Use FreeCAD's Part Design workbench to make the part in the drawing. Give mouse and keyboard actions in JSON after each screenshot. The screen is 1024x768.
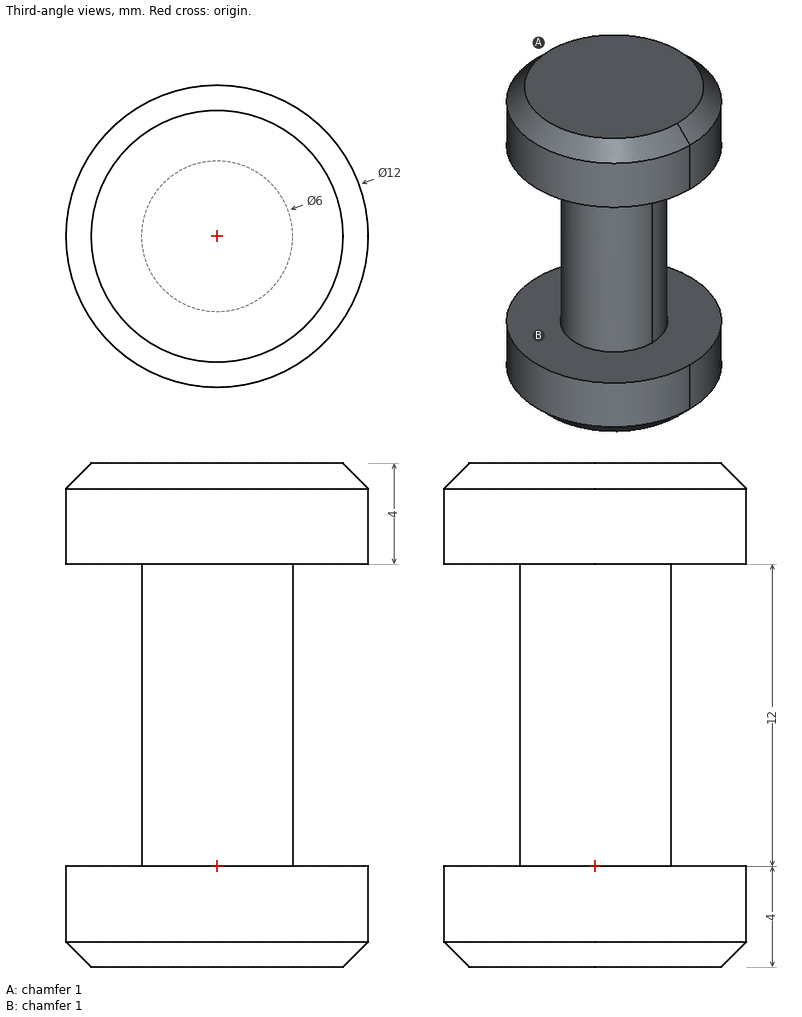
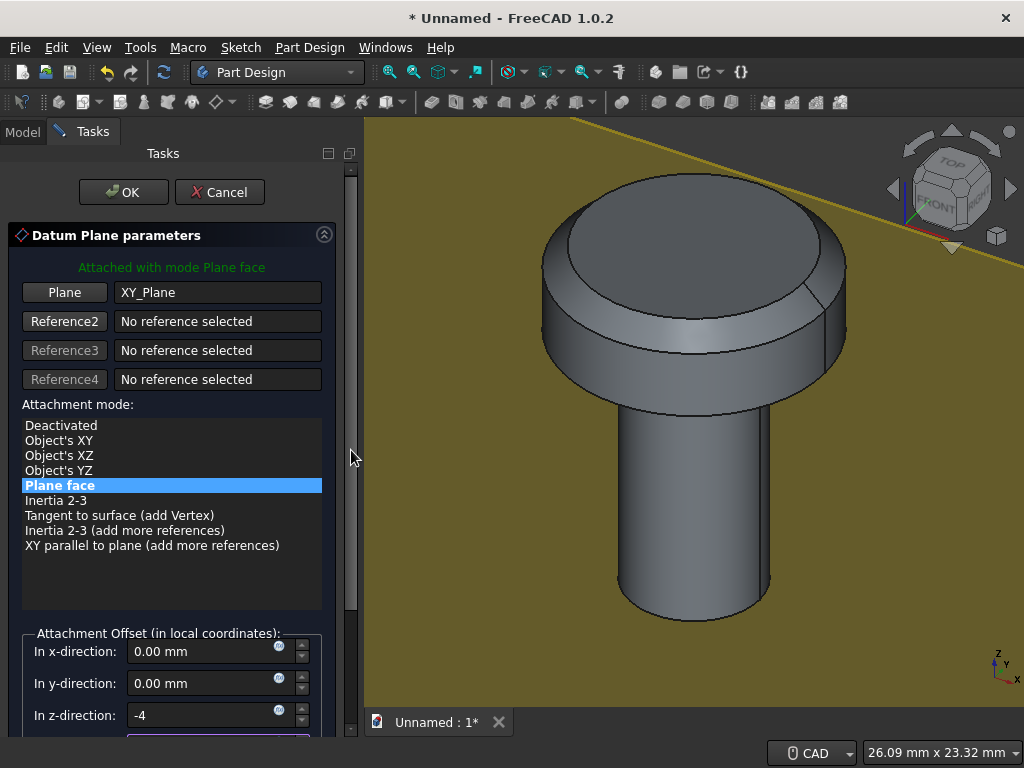
{"action": "left_click", "coordinate": [124, 192]}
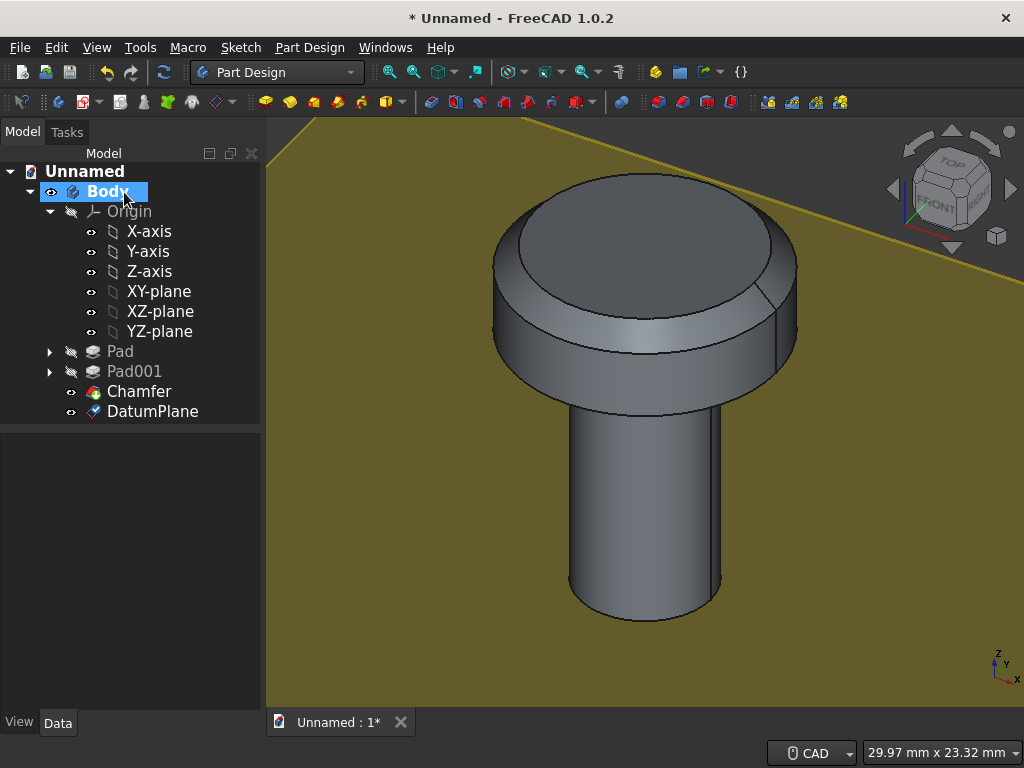
{"action": "left_click", "coordinate": [116, 412]}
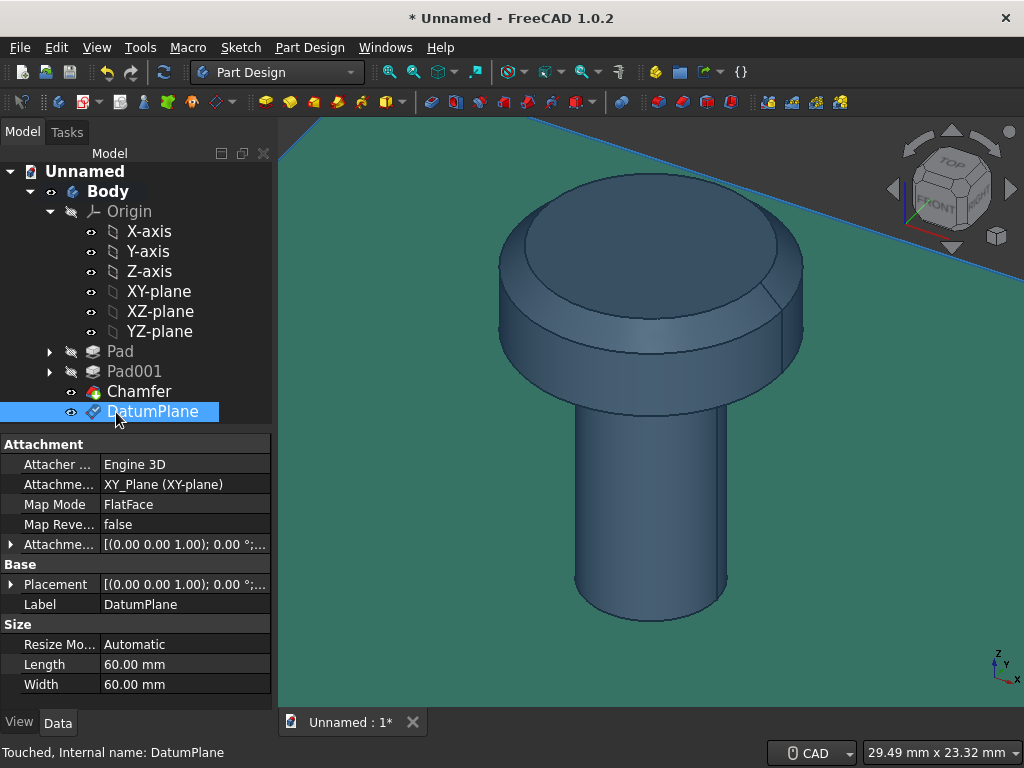
{"action": "left_click", "coordinate": [84, 102]}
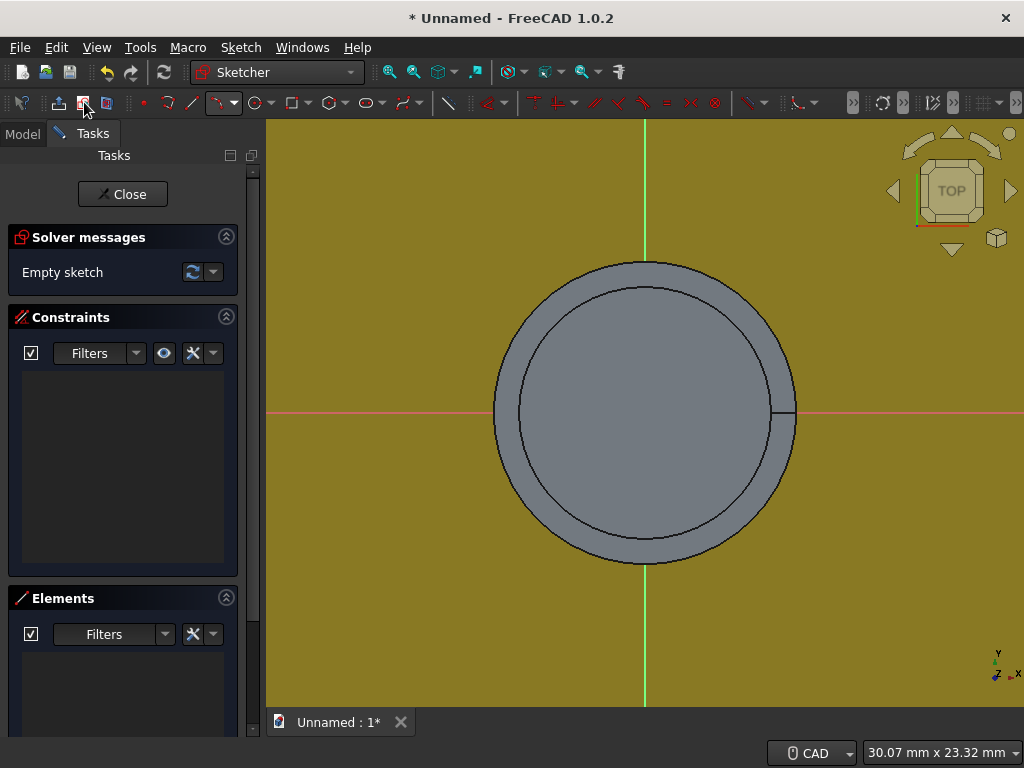
{"action": "key", "text": "q s"}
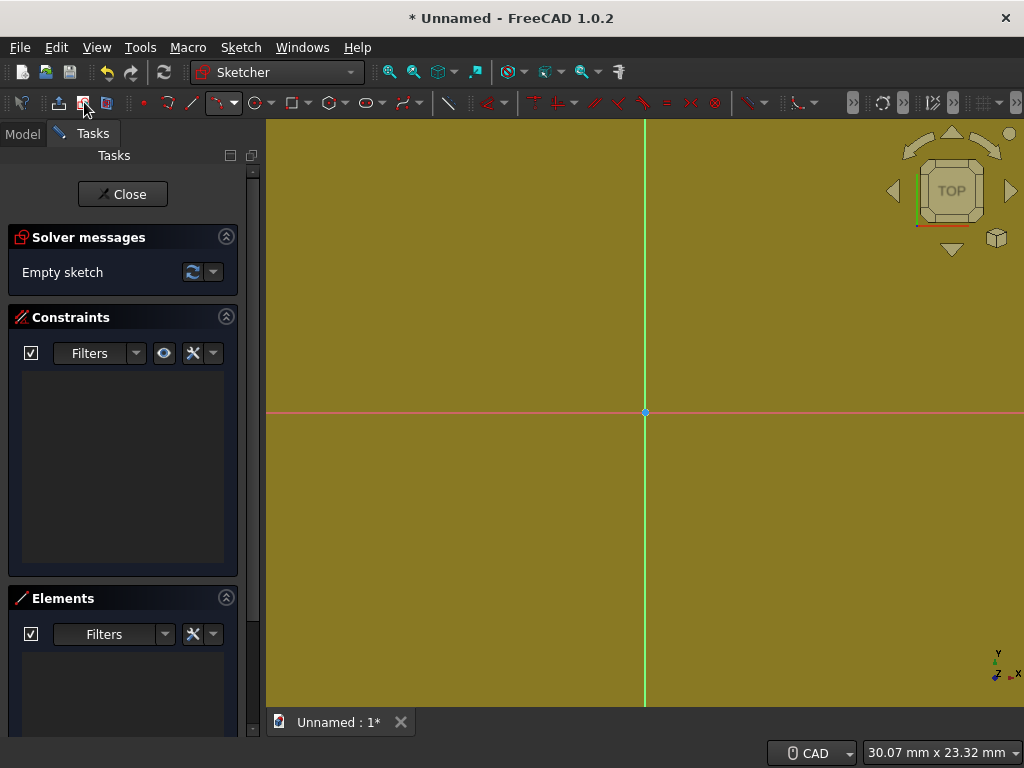
{"action": "key", "text": "g c"}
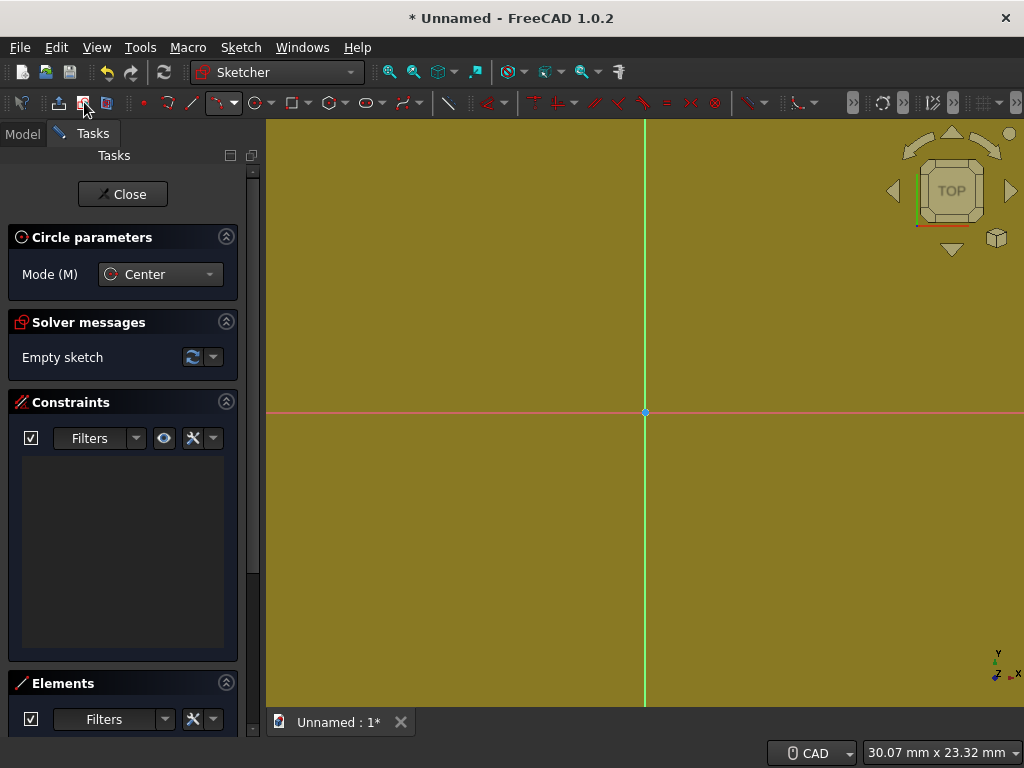
{"action": "left_click", "coordinate": [645, 413]}
{"action": "left_click", "coordinate": [752, 306]}
{"action": "key", "text": "Escape"}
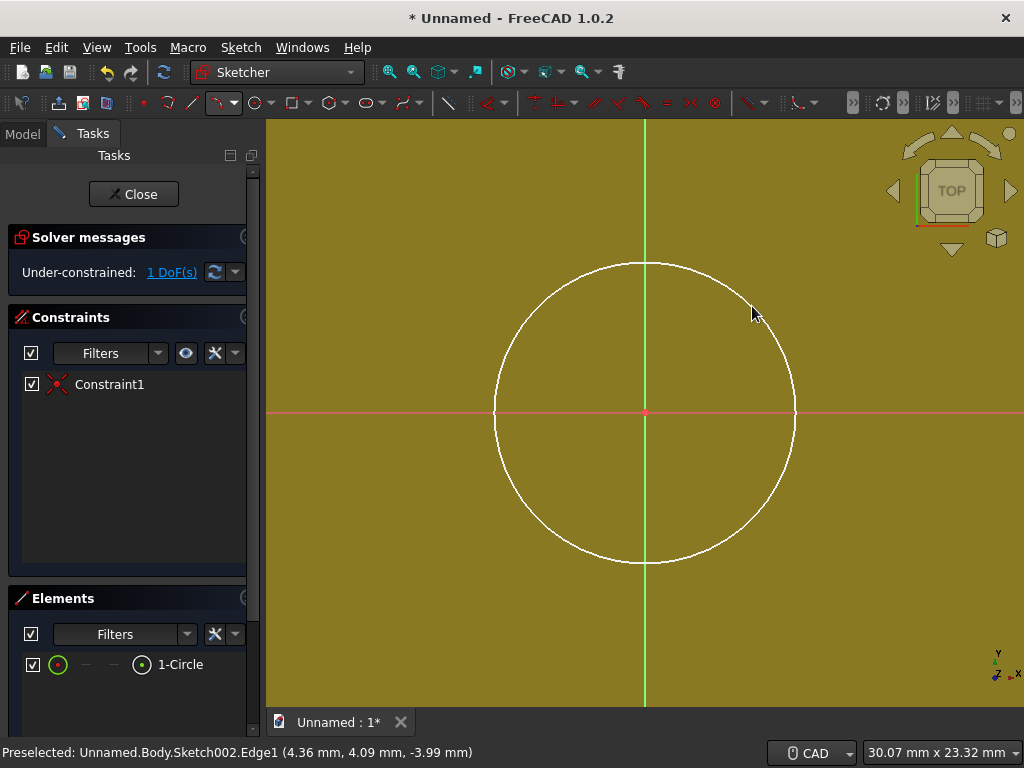
{"action": "left_click", "coordinate": [488, 104]}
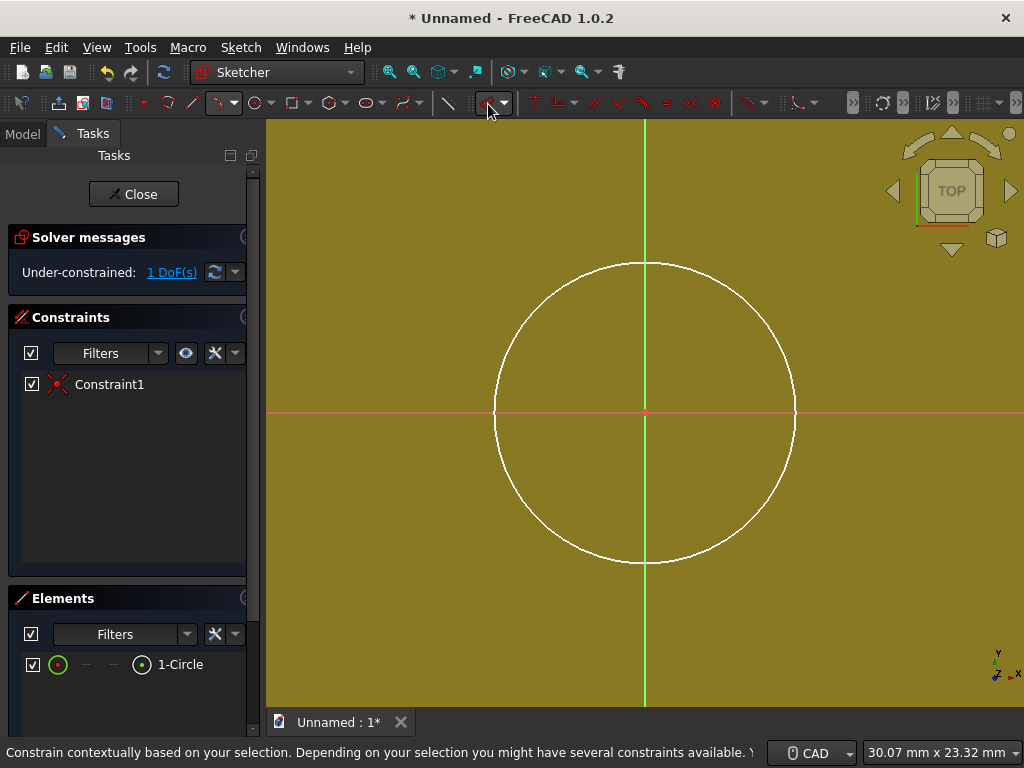
{"action": "left_click", "coordinate": [751, 306]}
{"action": "left_click", "coordinate": [774, 283]}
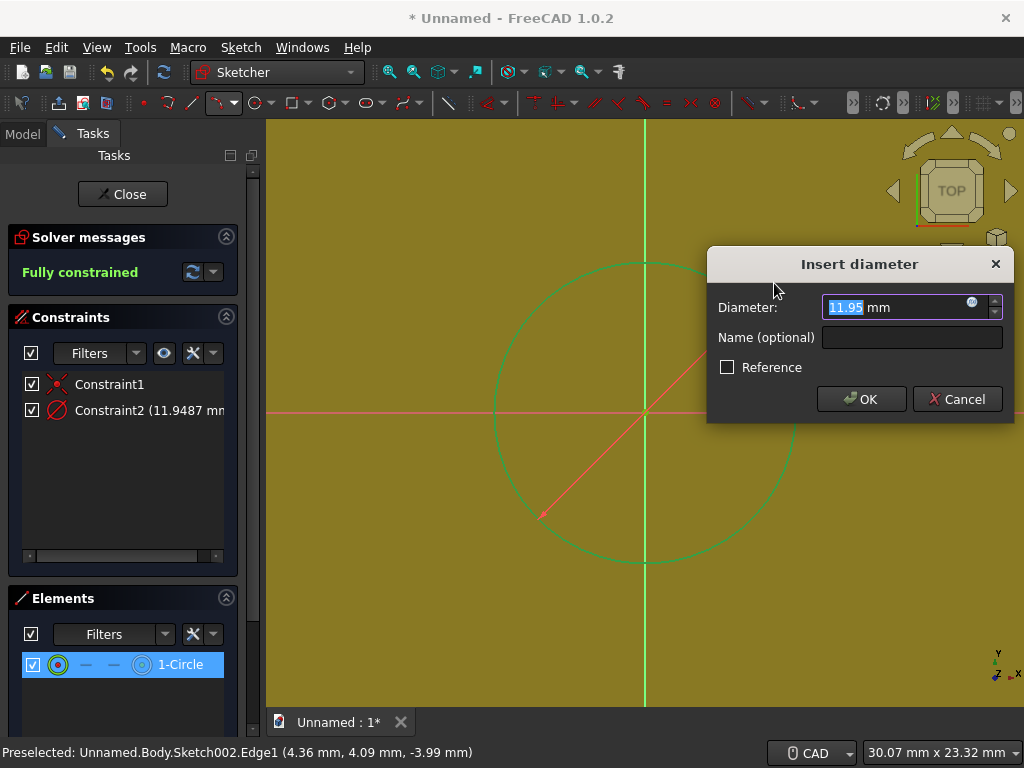
{"action": "type", "text": "12"}
{"action": "key", "text": "Return"}
{"action": "key", "text": "Escape"}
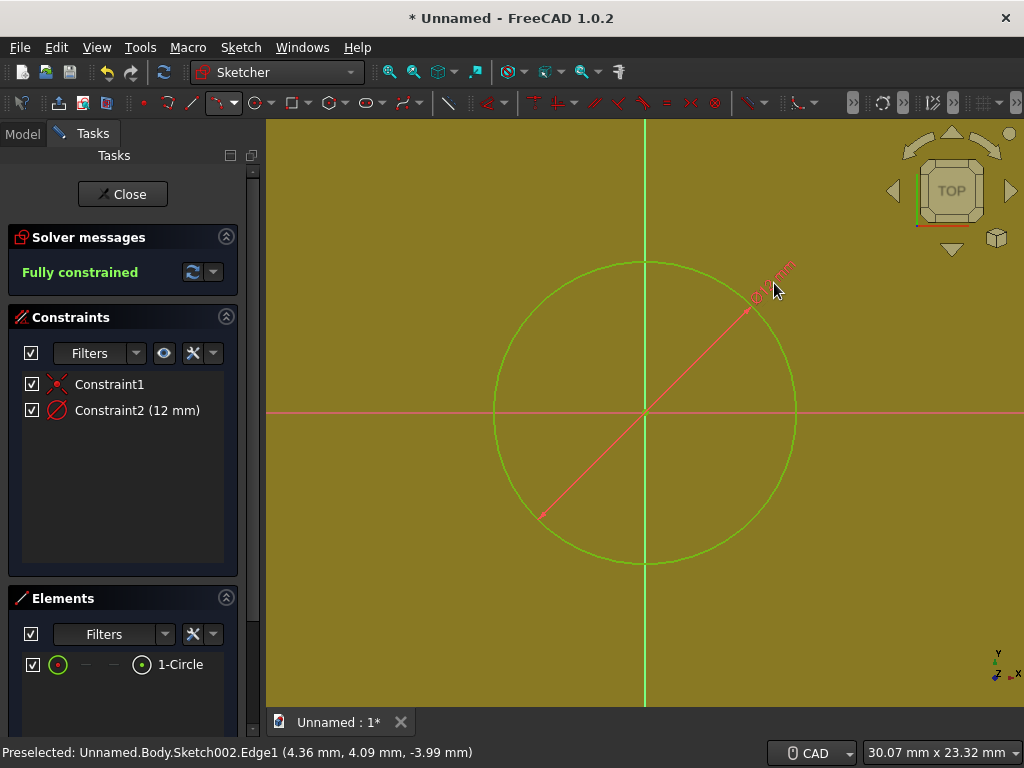
{"action": "left_click", "coordinate": [123, 194]}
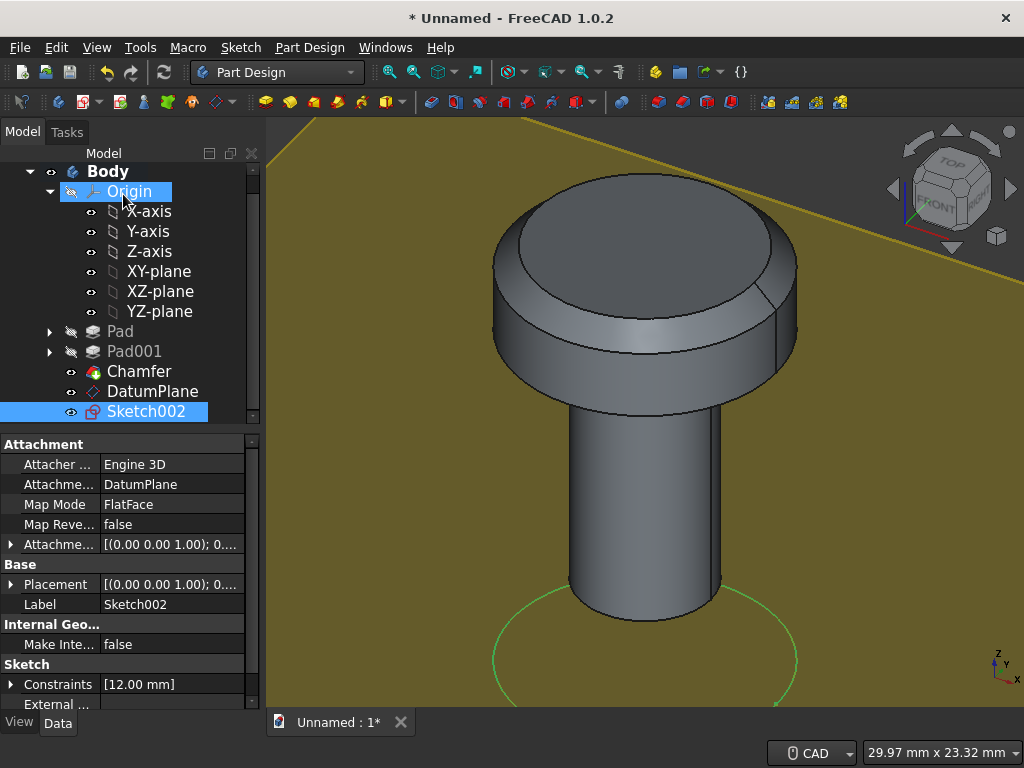
{"action": "left_click", "coordinate": [266, 102]}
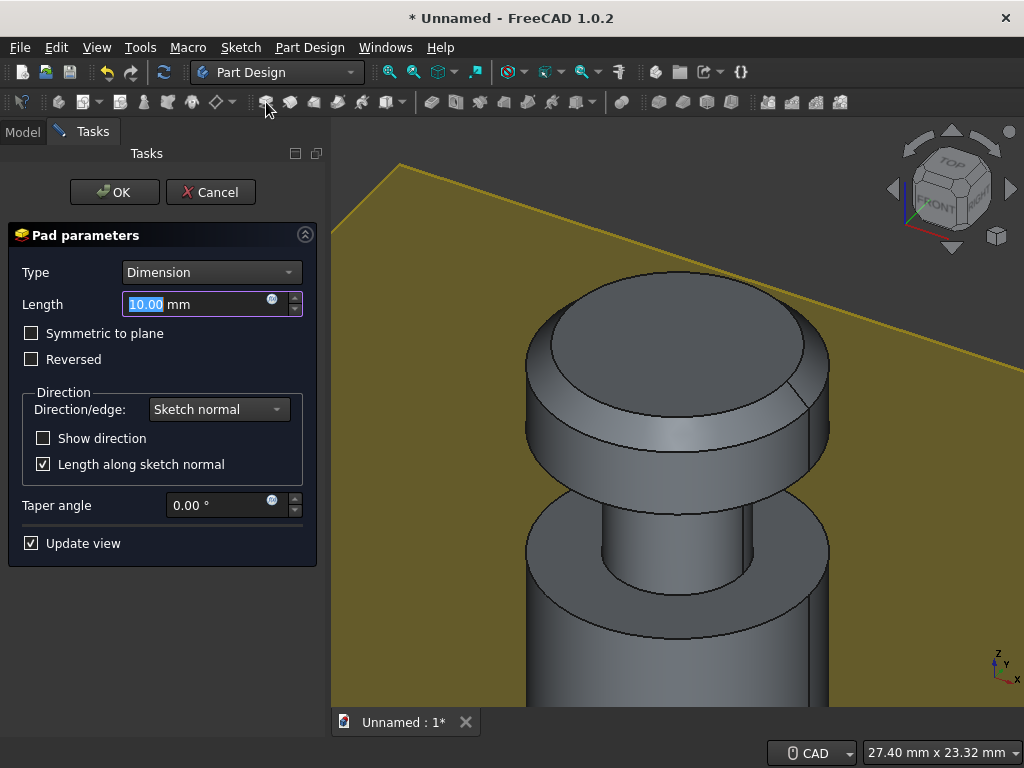
{"action": "type", "text": "4"}
{"action": "key", "text": "Tab"}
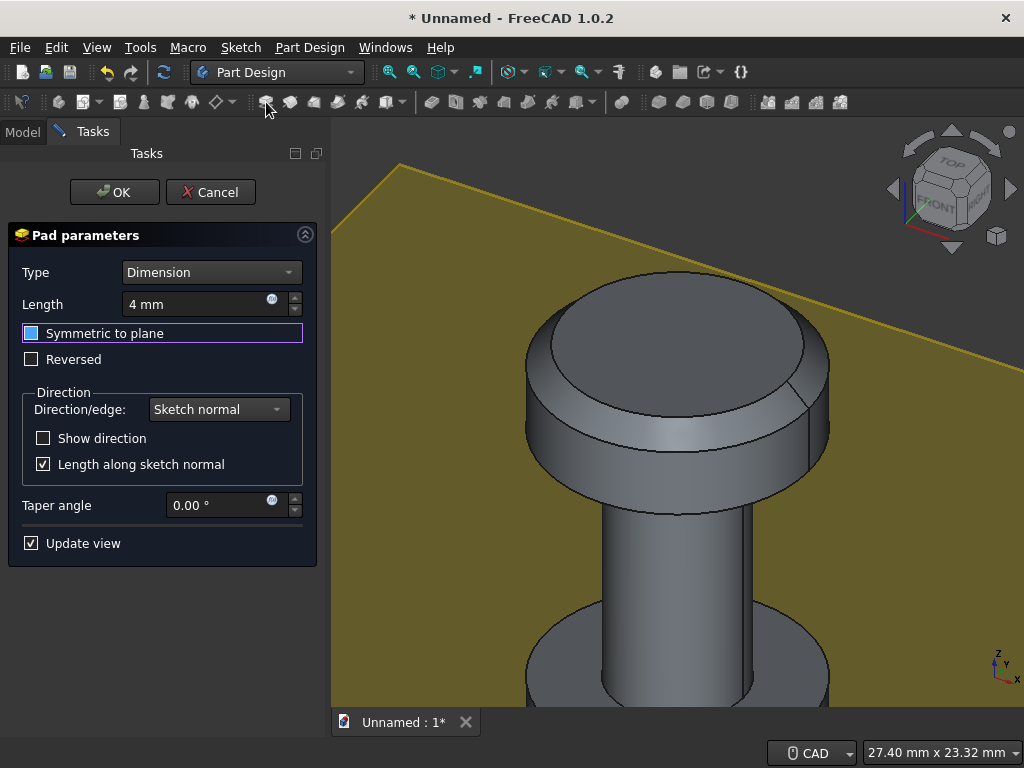
{"action": "left_click", "coordinate": [115, 192]}